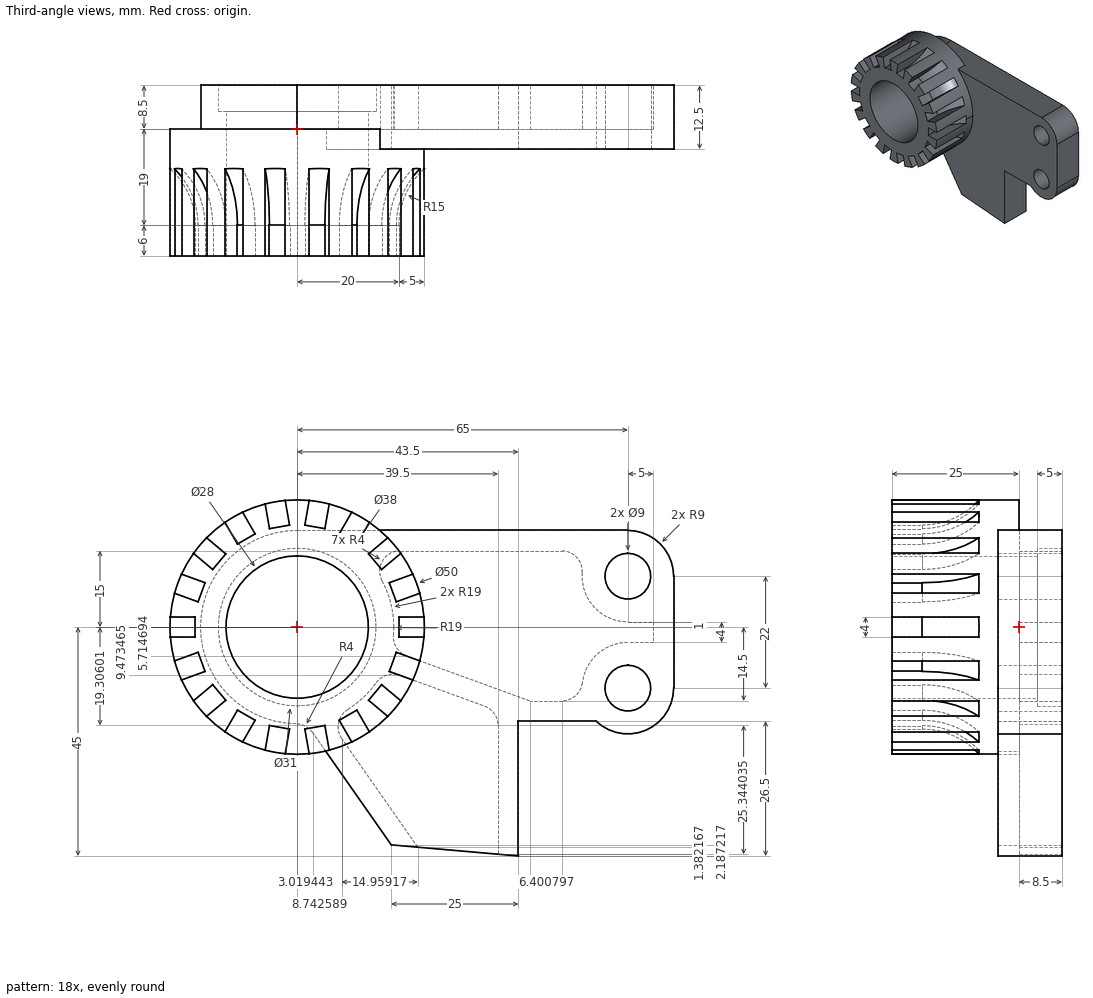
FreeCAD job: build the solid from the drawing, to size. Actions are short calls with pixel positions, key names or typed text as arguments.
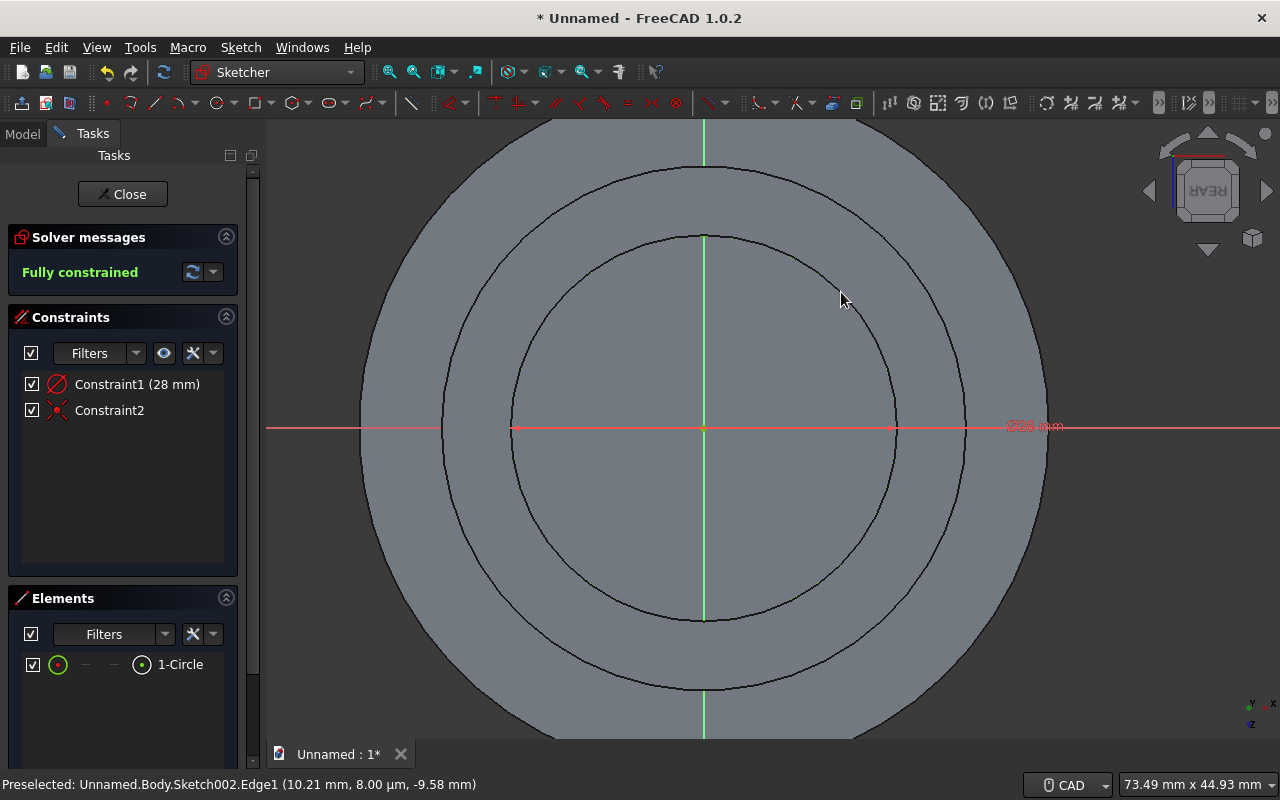
click(123, 194)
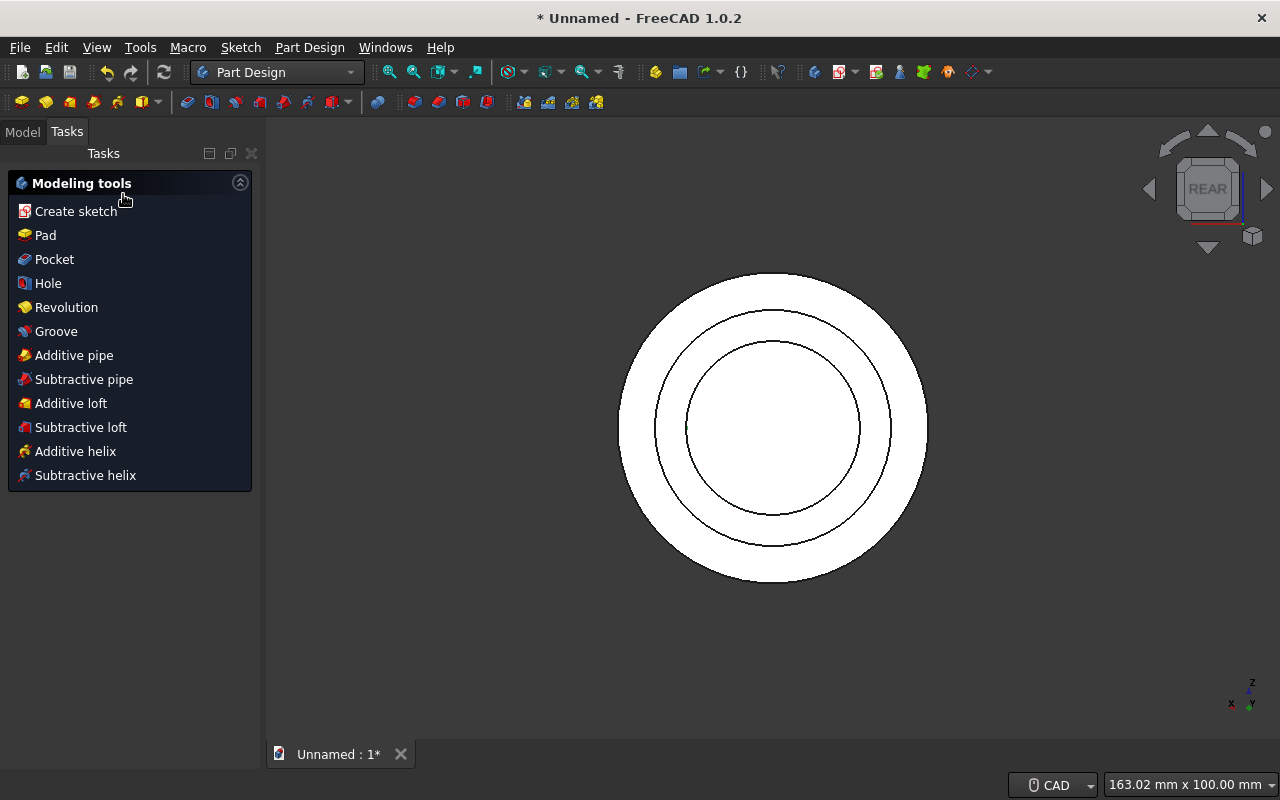
click(188, 102)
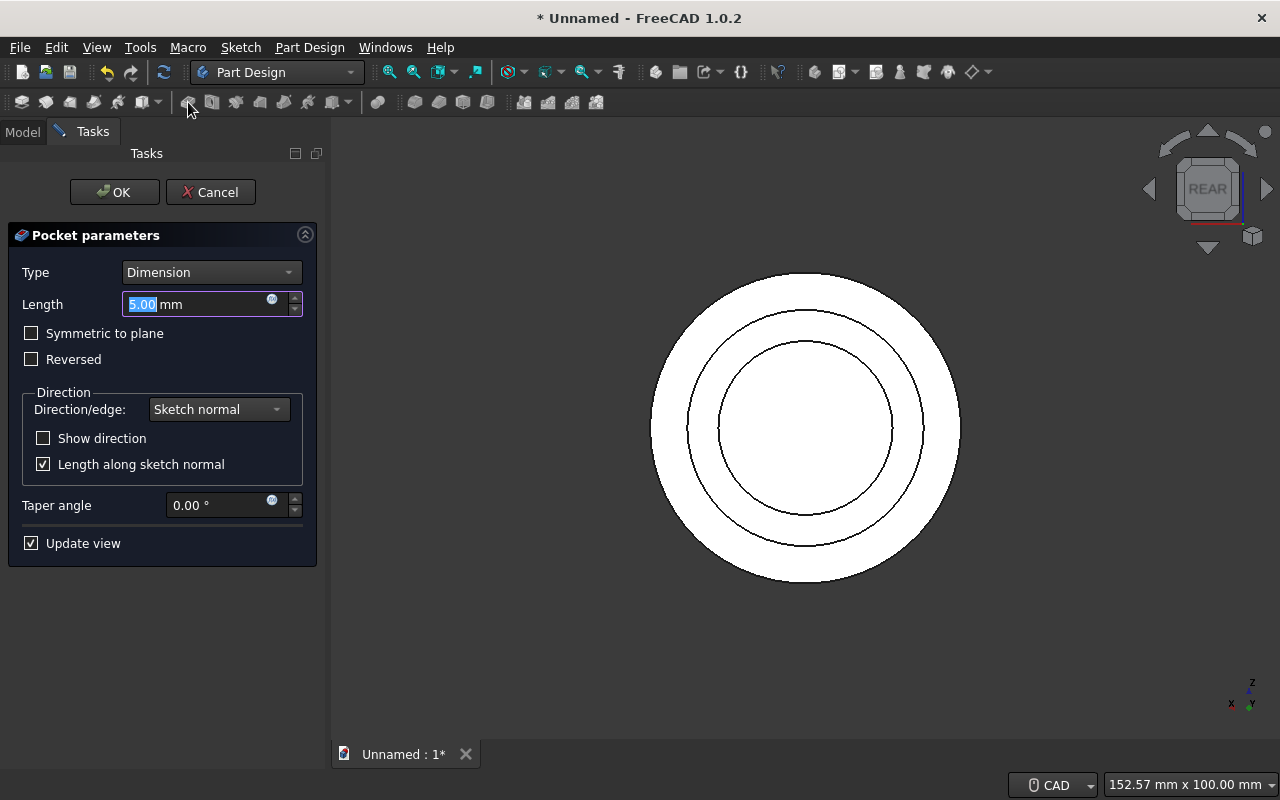
click(212, 272)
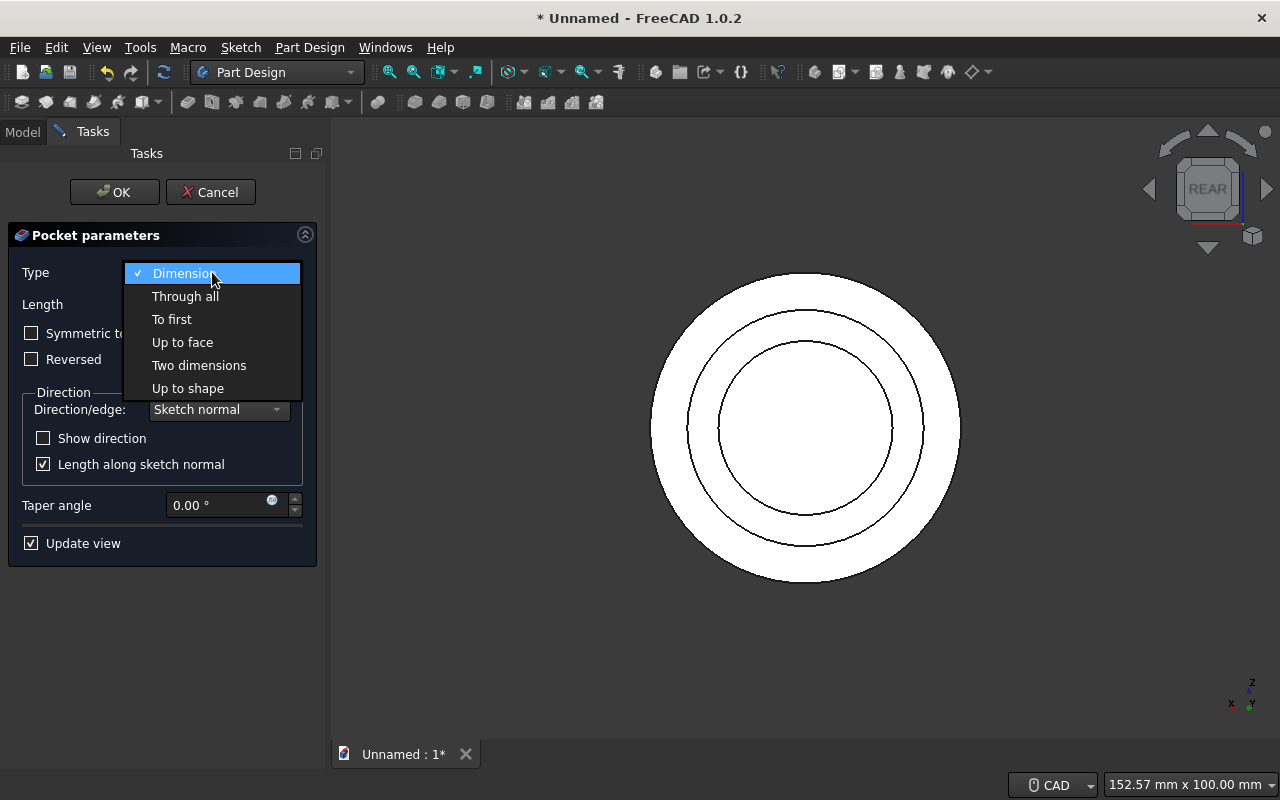
click(212, 320)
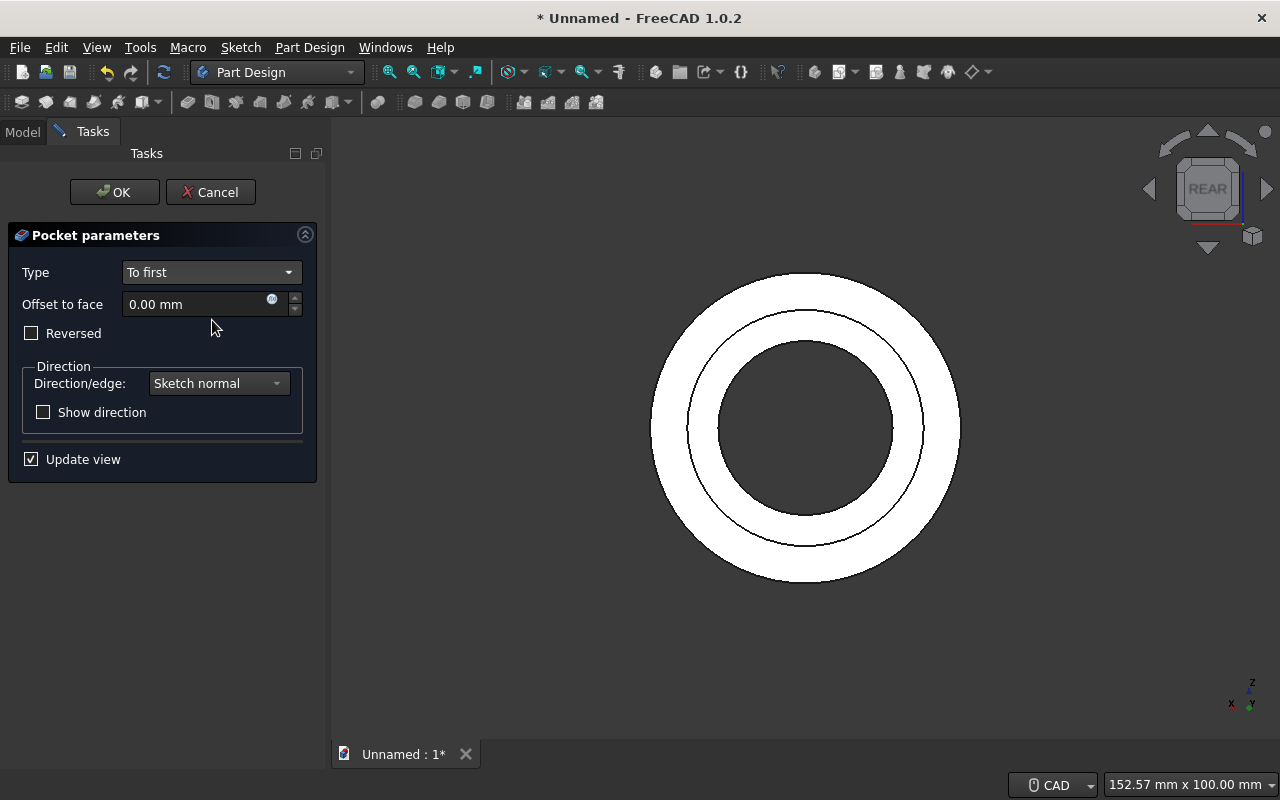
click(115, 192)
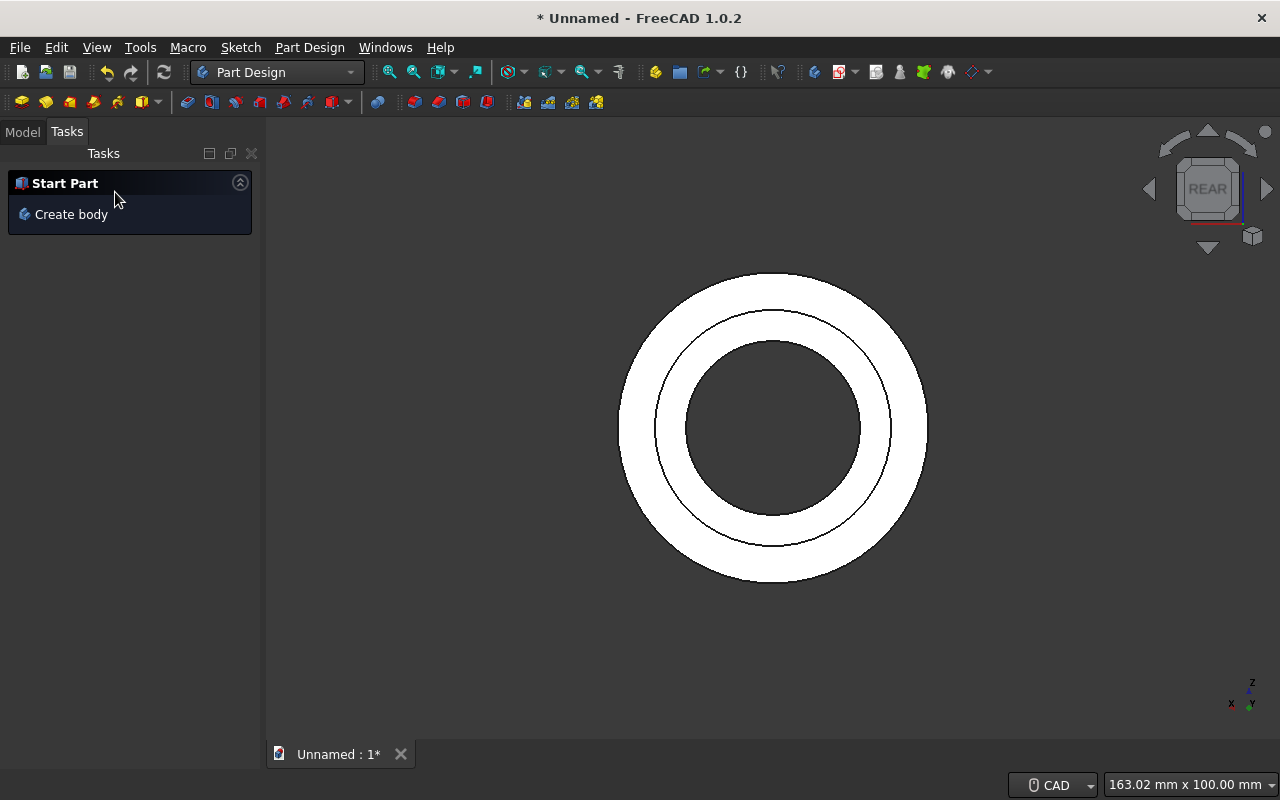
click(773, 326)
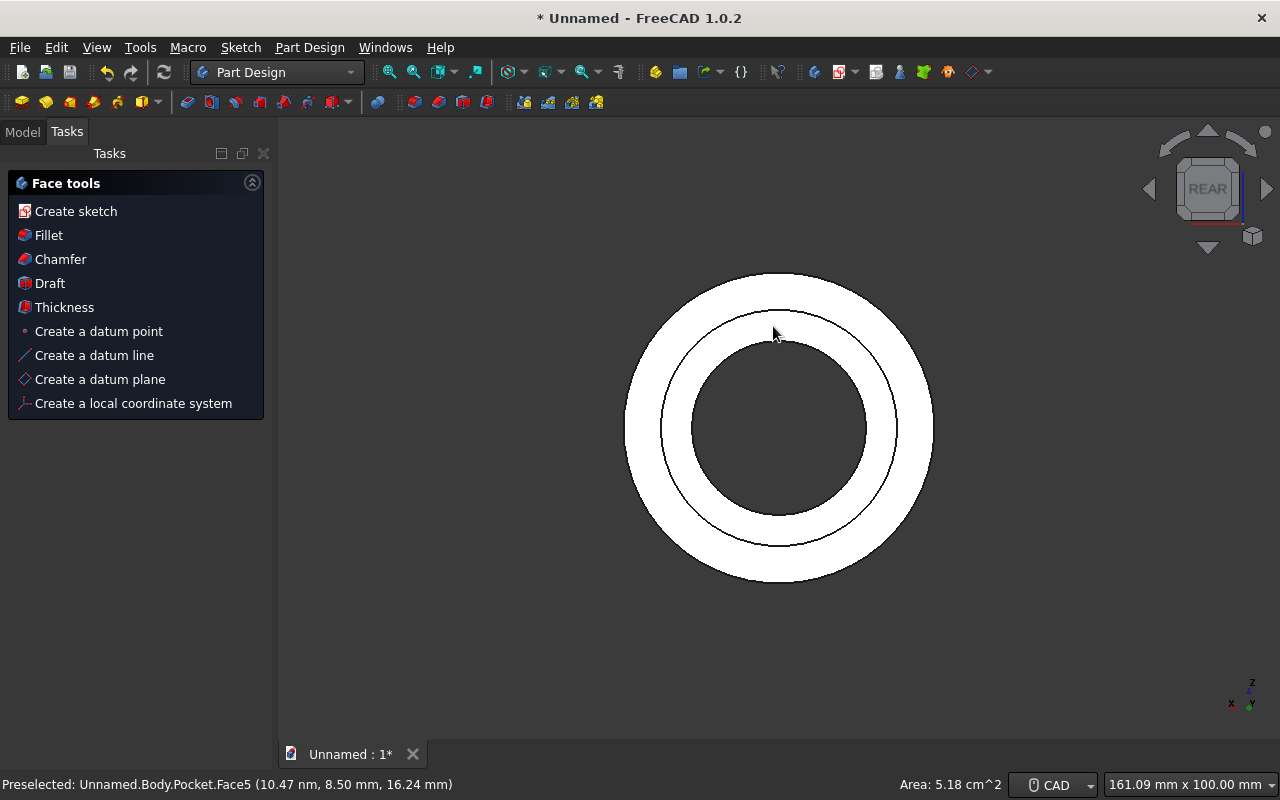
click(840, 72)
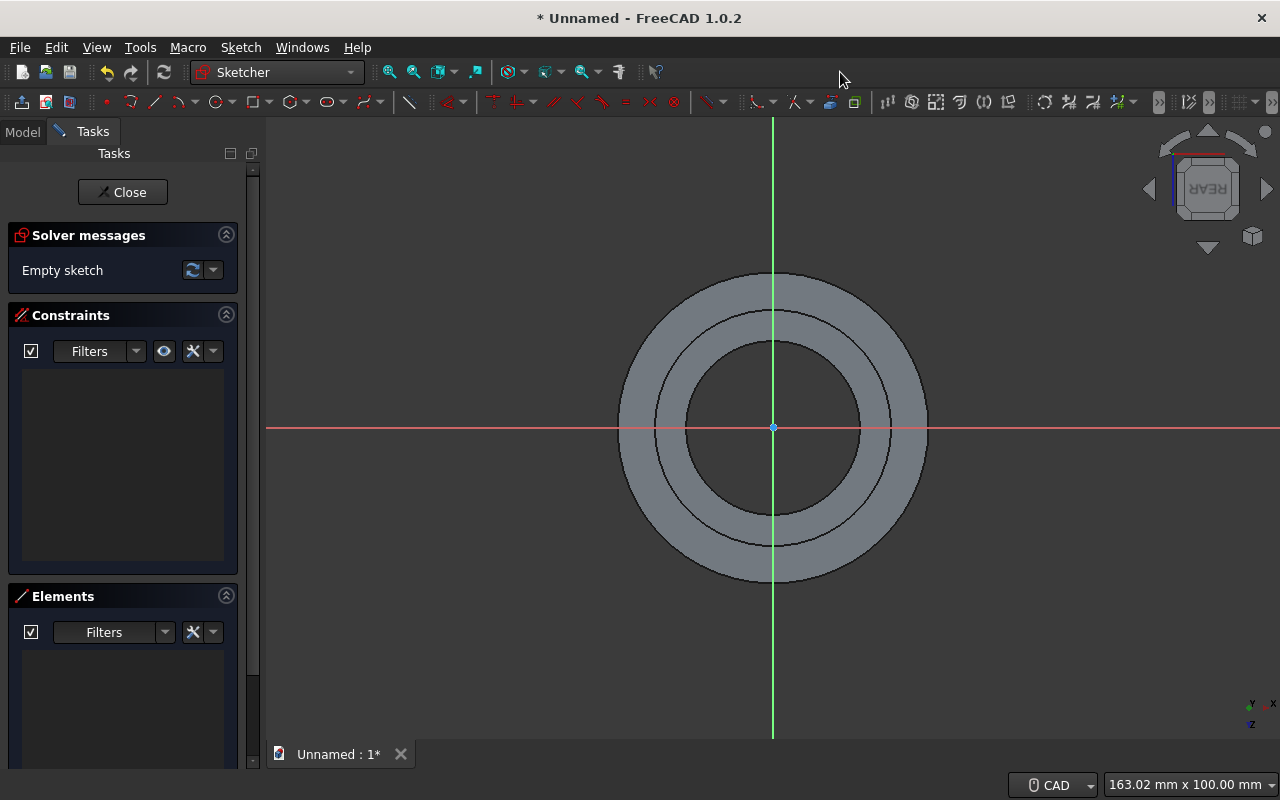
scroll(829, 428, up, 4)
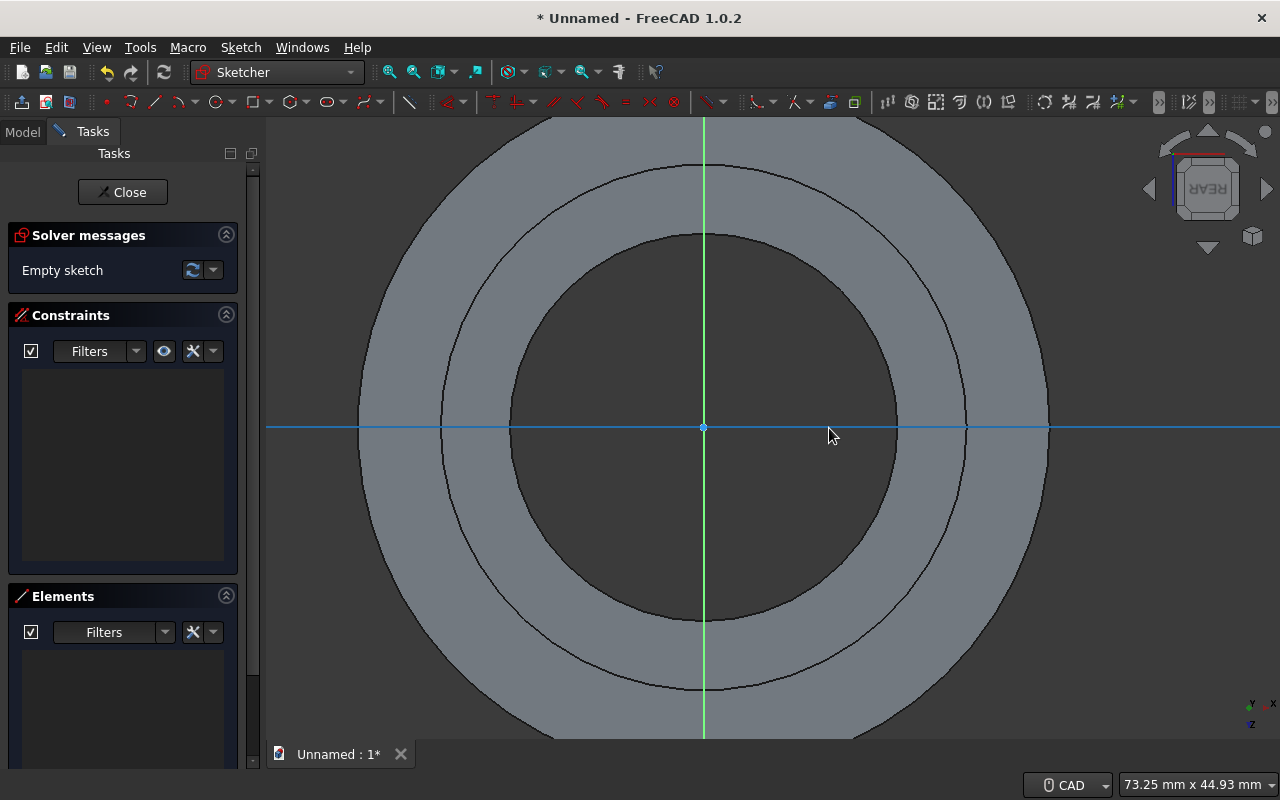
click(216, 102)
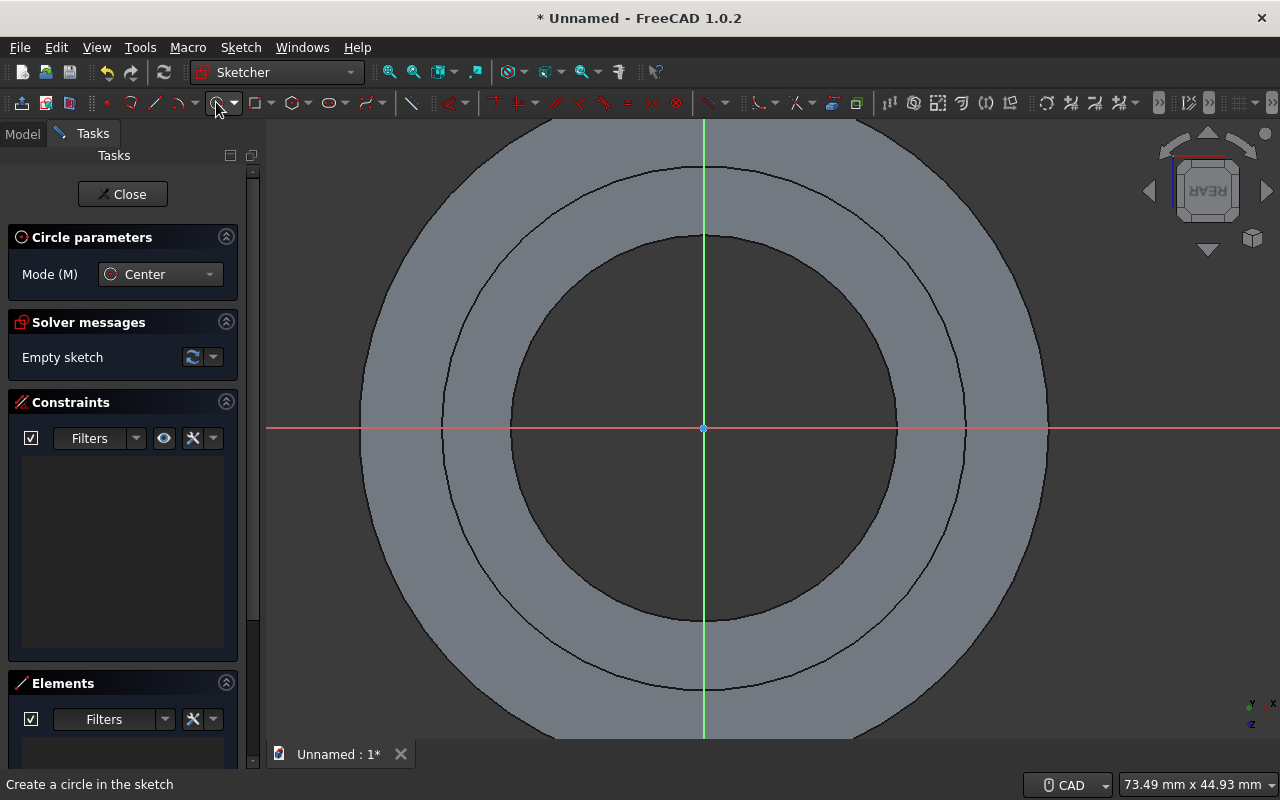
click(704, 428)
move(855, 277)